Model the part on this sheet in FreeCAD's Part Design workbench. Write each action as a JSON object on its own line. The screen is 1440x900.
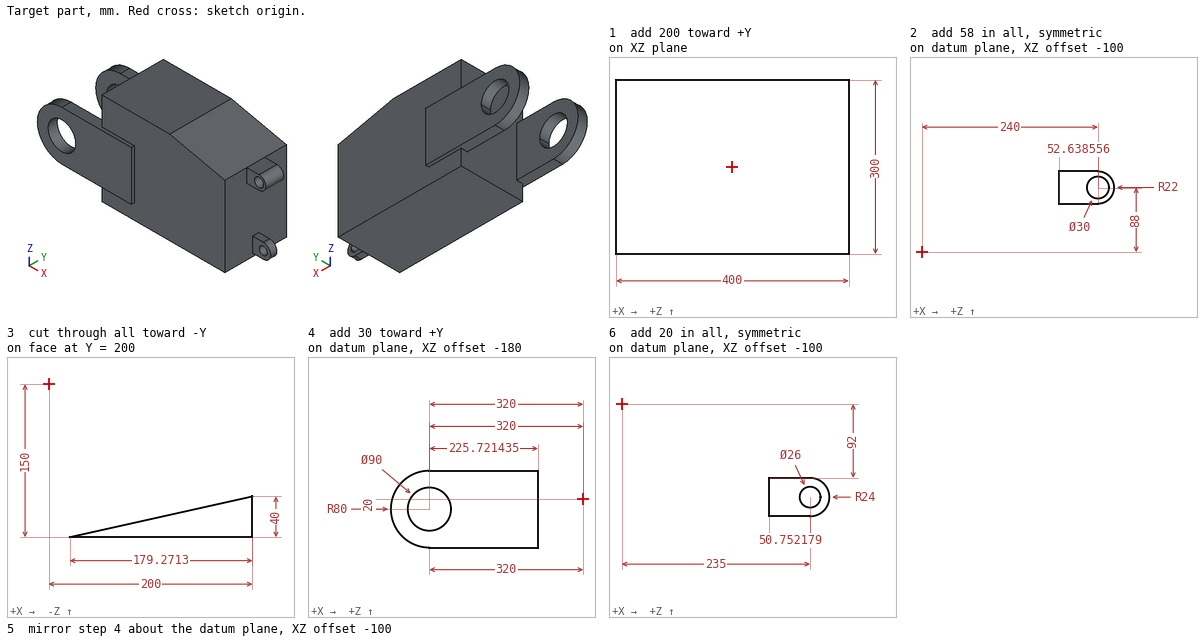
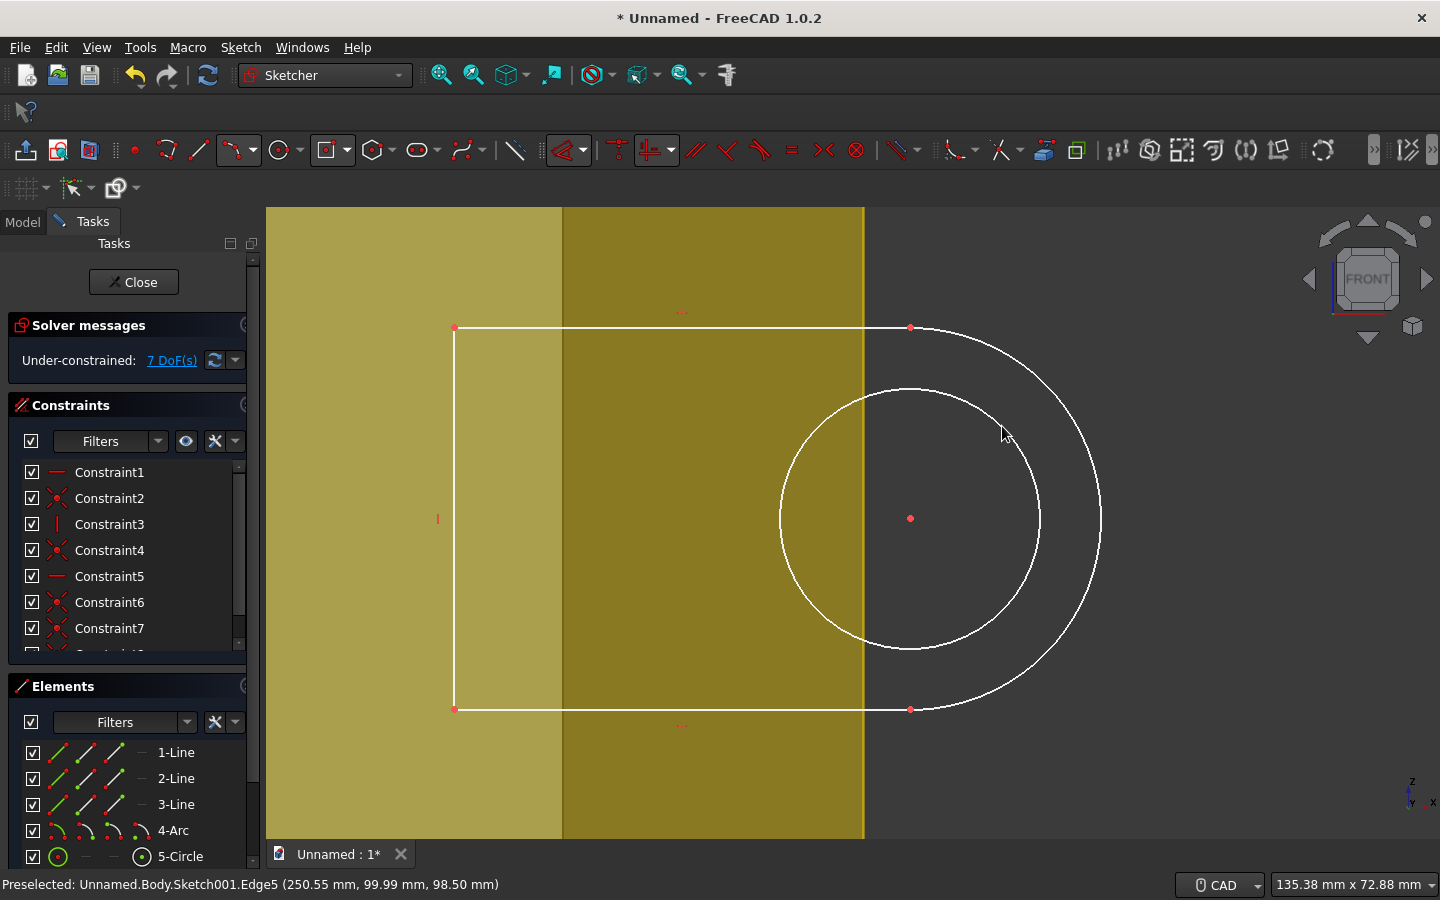
{"action": "left_click", "coordinate": [773, 710]}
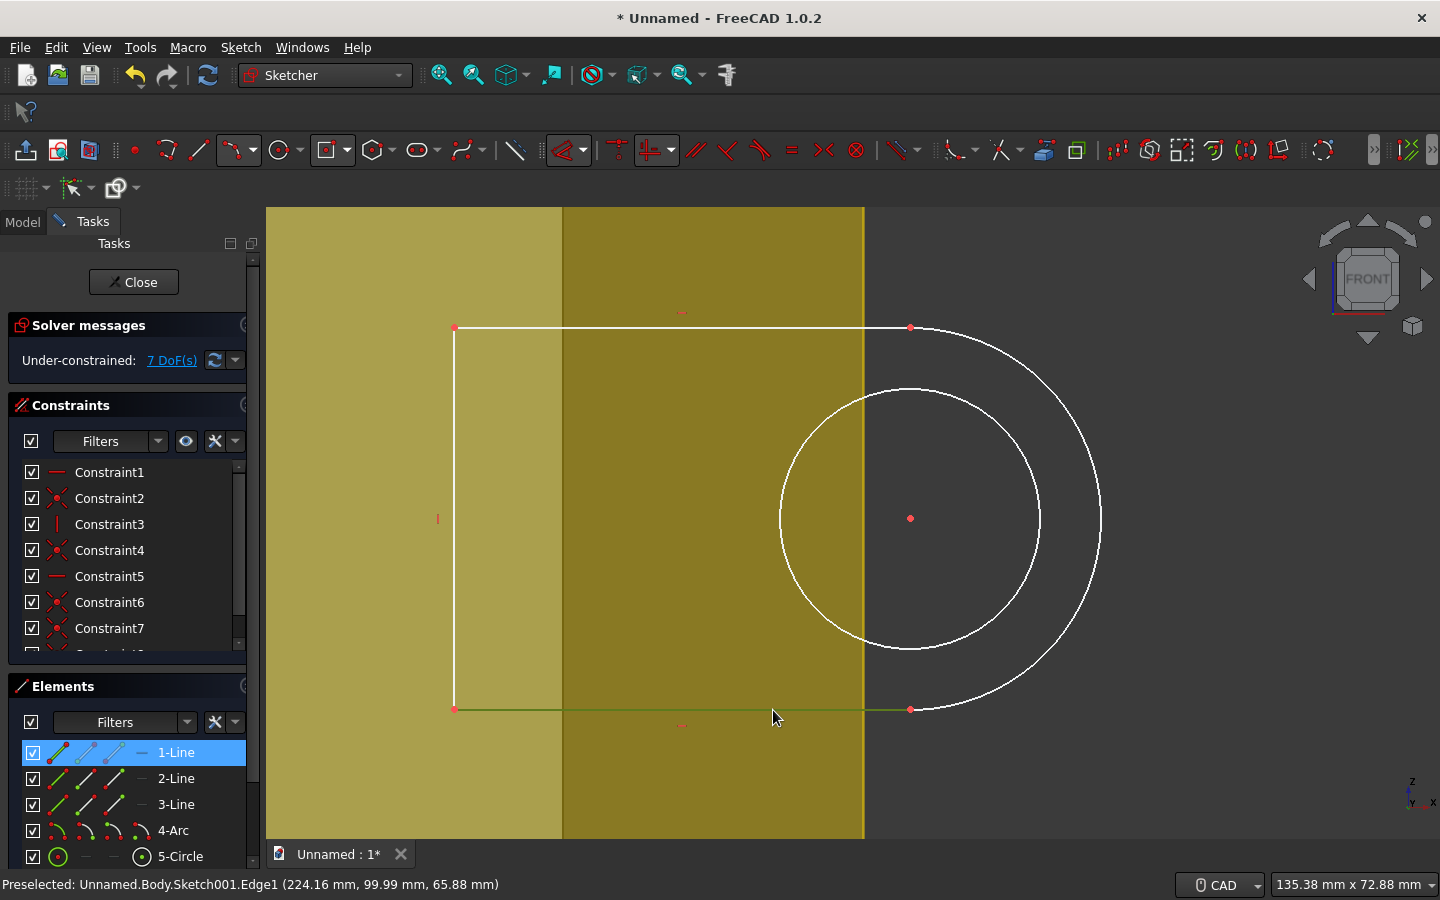
{"action": "left_click", "coordinate": [1065, 631]}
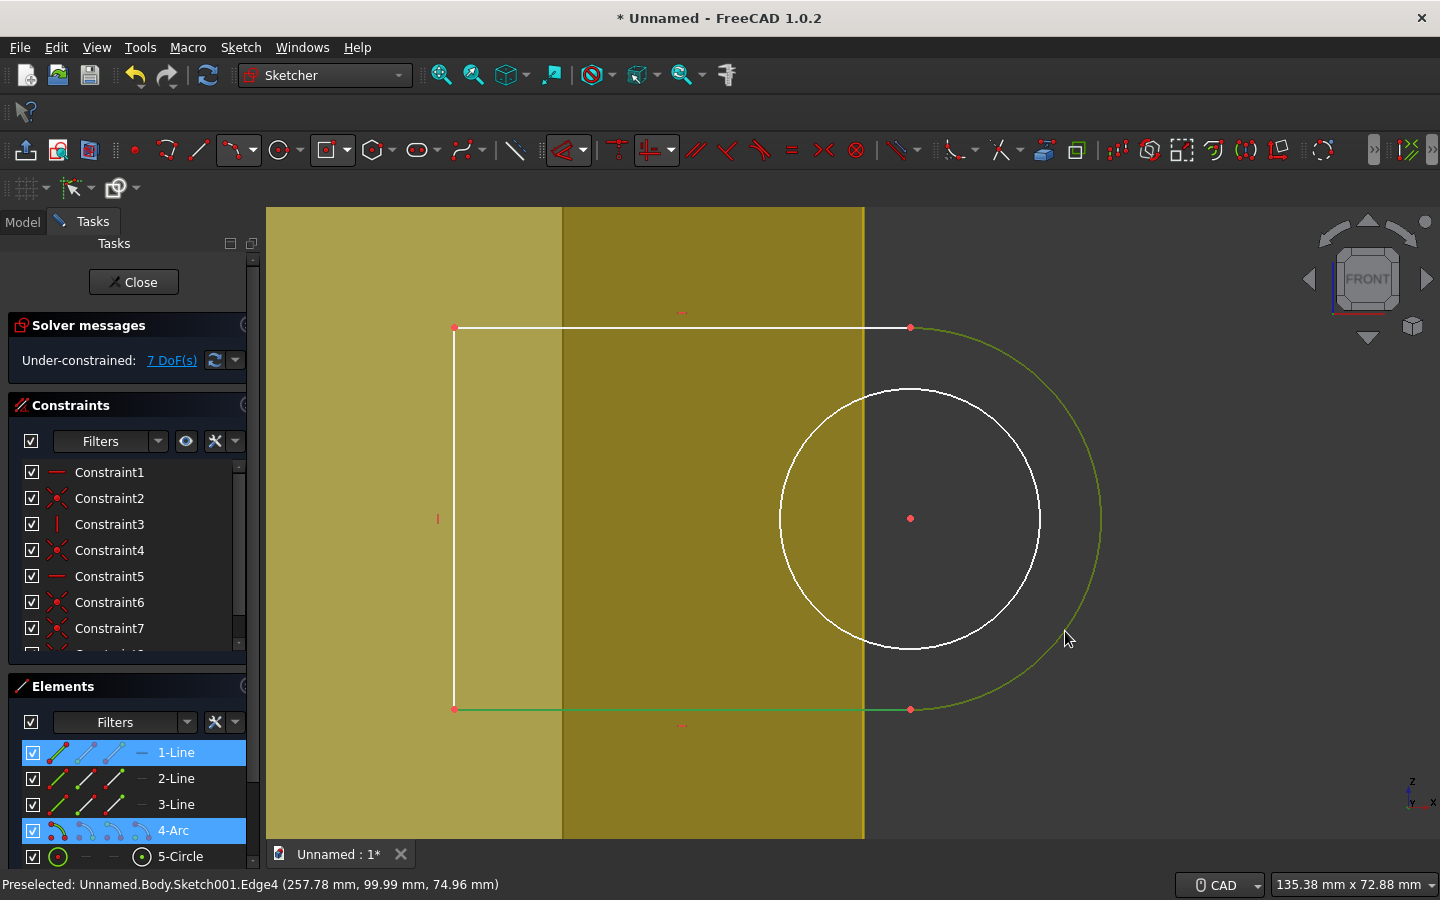
{"action": "left_click", "coordinate": [760, 150]}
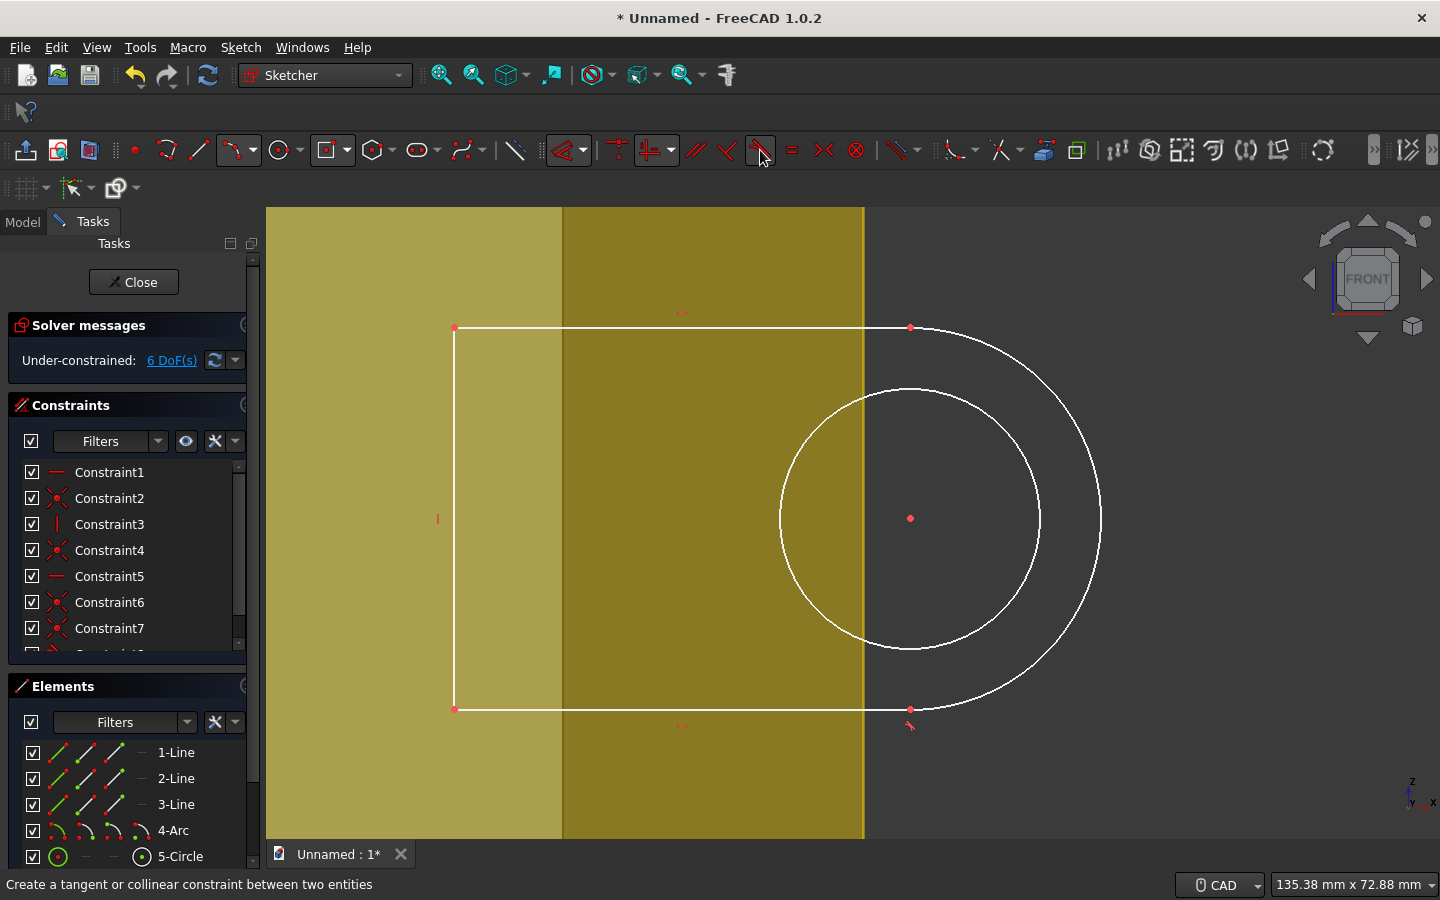
{"action": "left_click", "coordinate": [591, 328]}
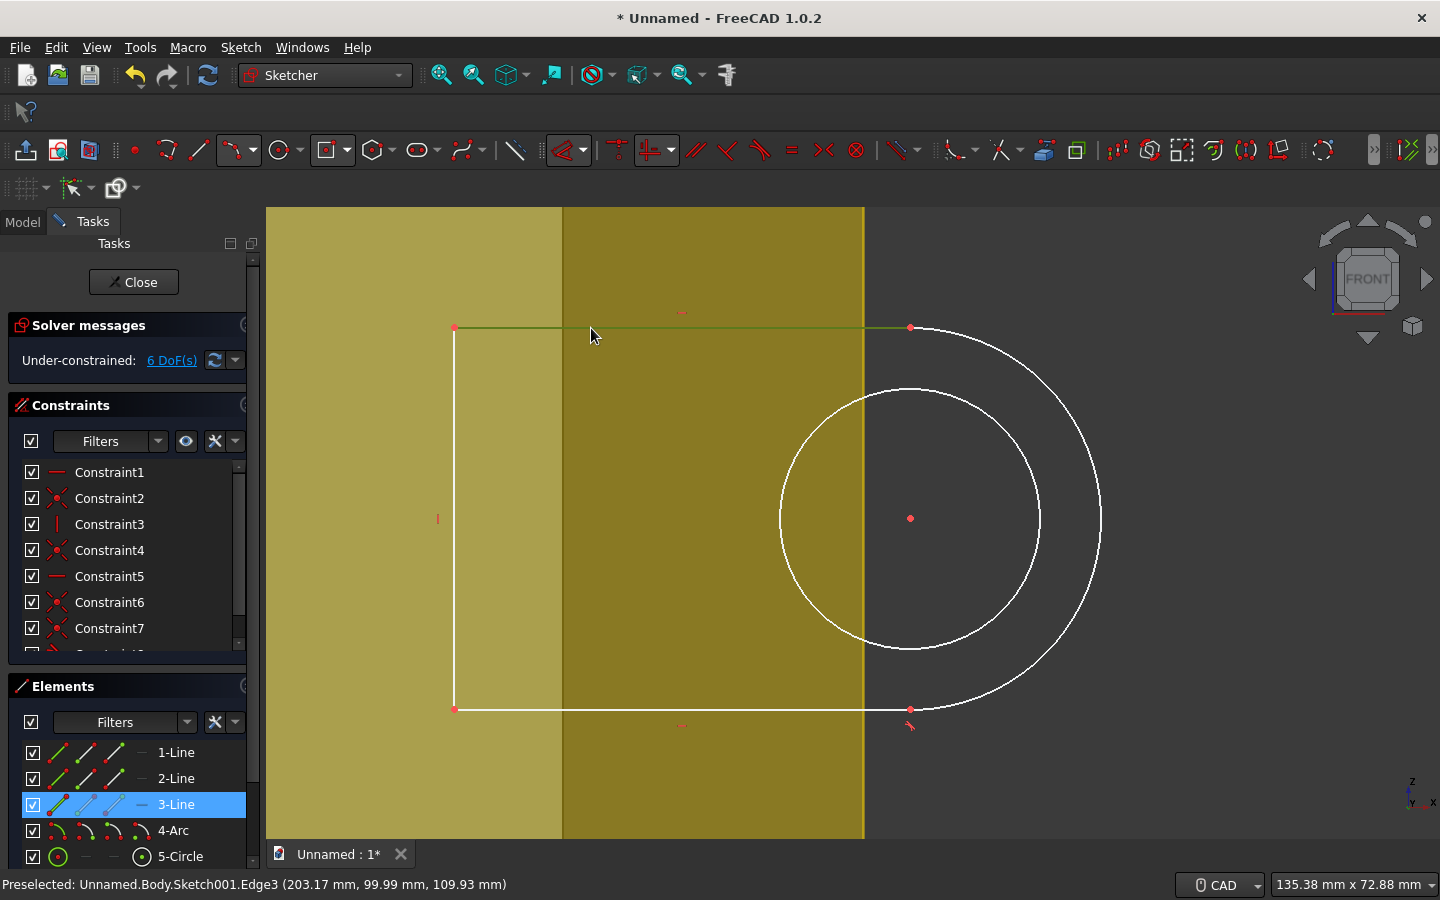
{"action": "left_click", "coordinate": [1065, 631]}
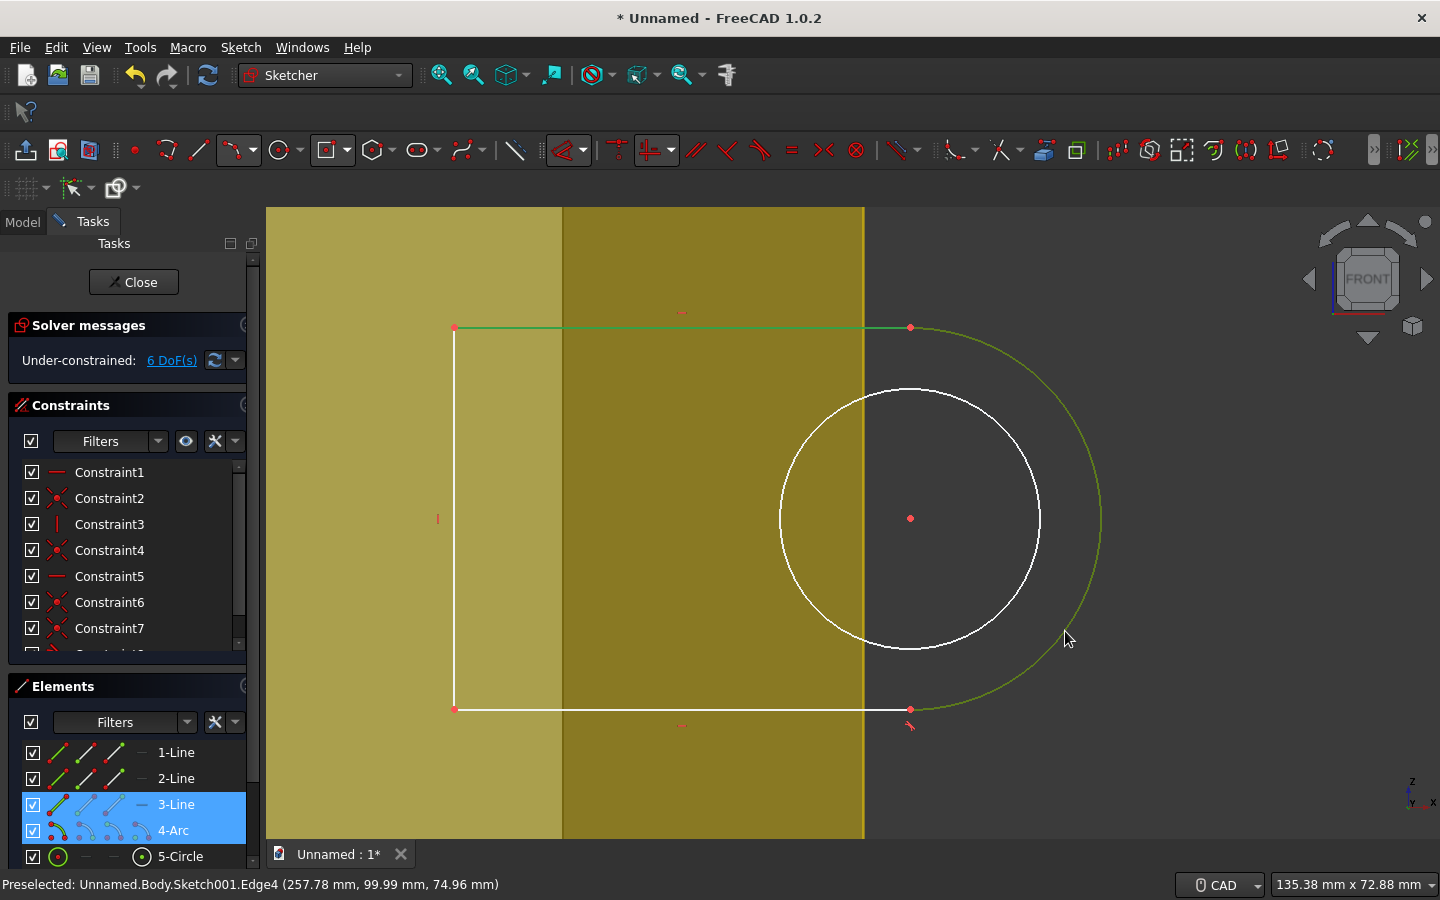
{"action": "left_click", "coordinate": [760, 150]}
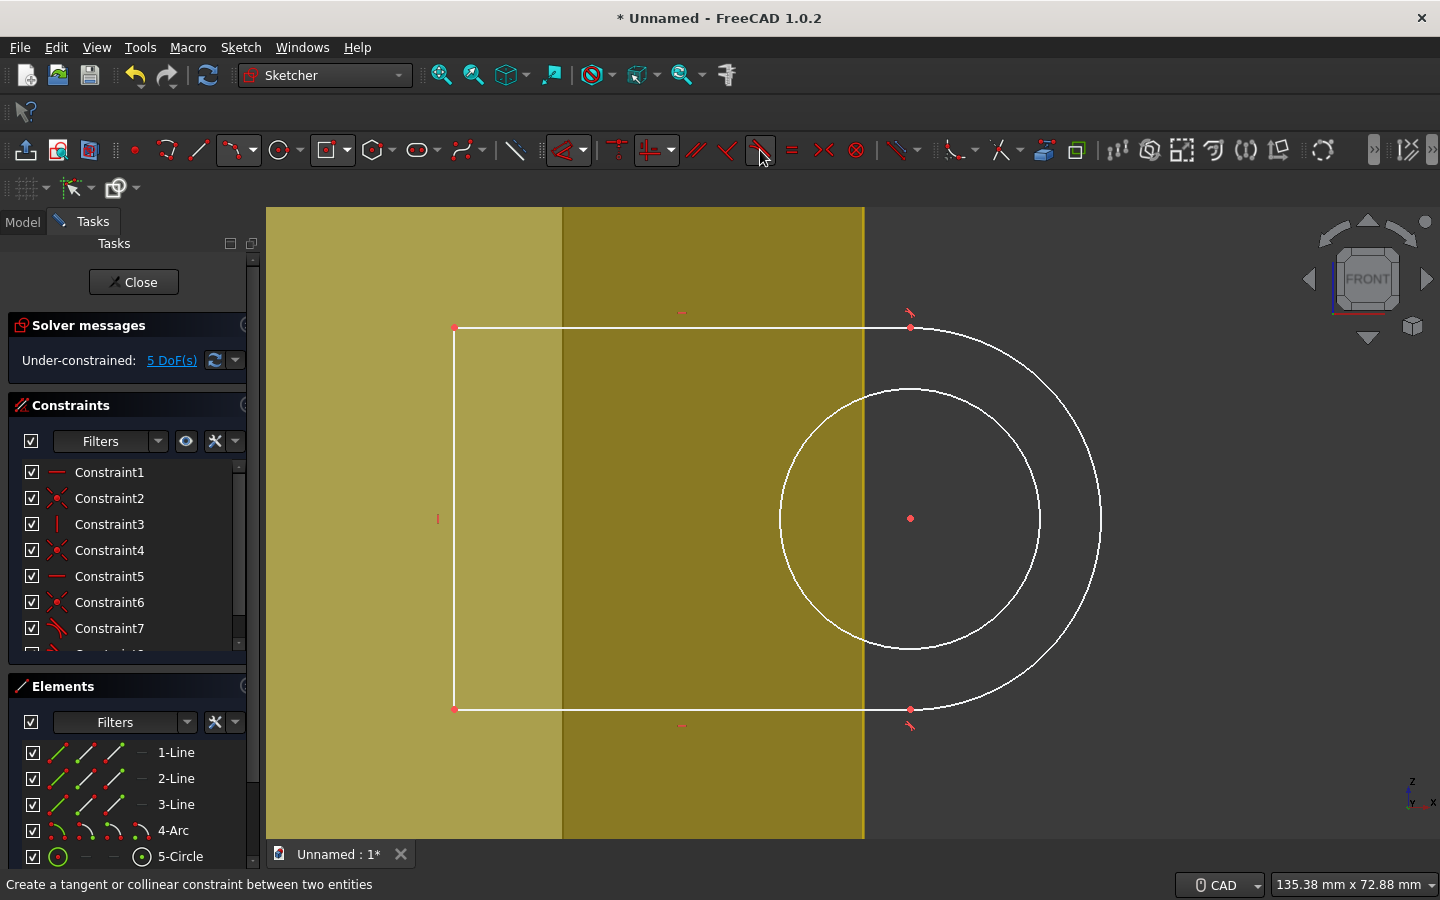
{"action": "left_click", "coordinate": [1065, 631]}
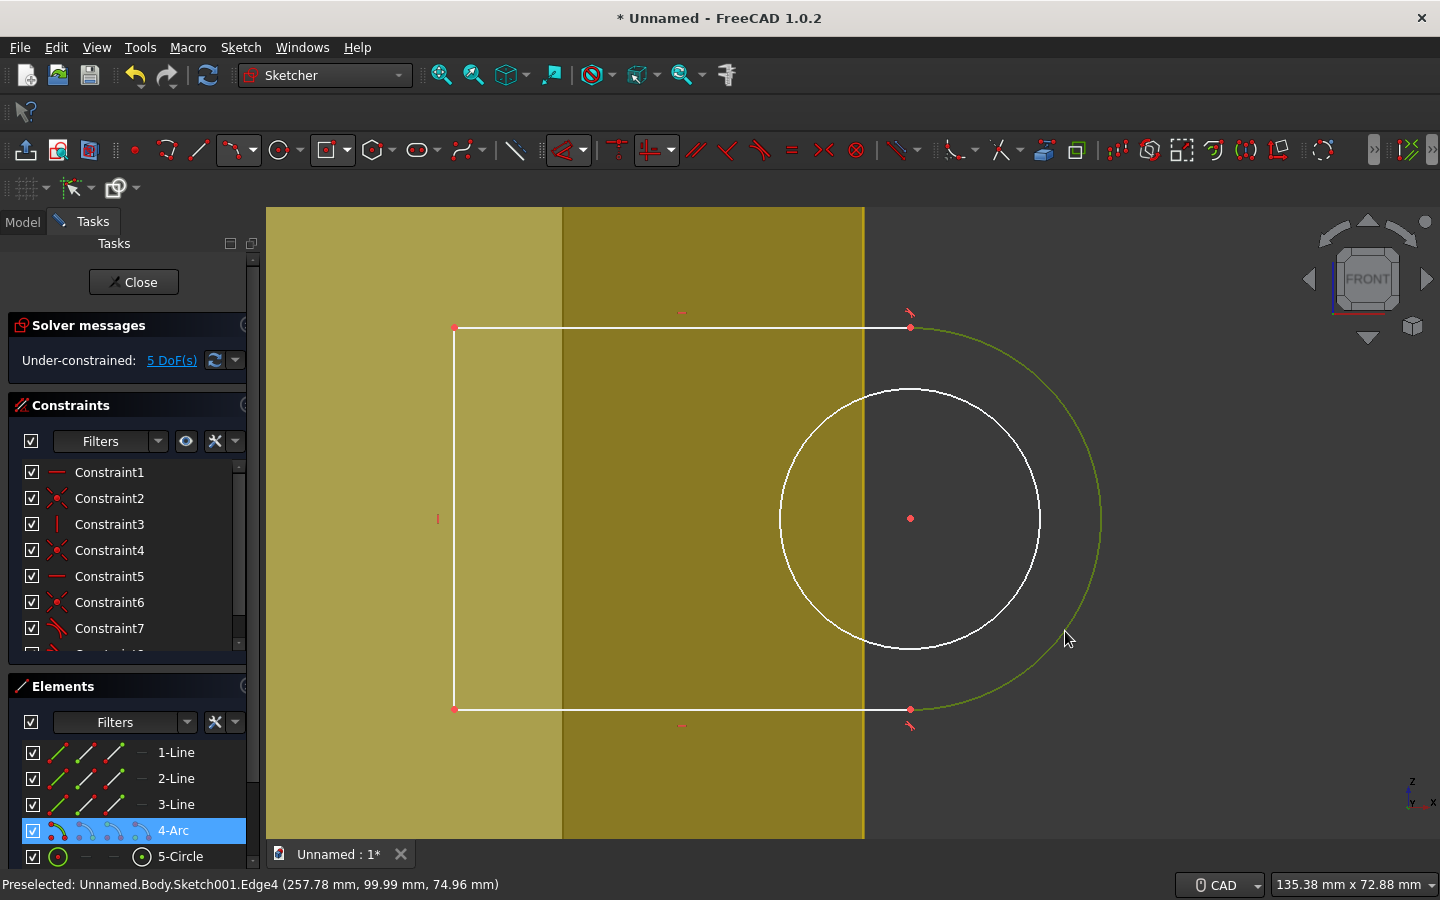
{"action": "left_click", "coordinate": [586, 150]}